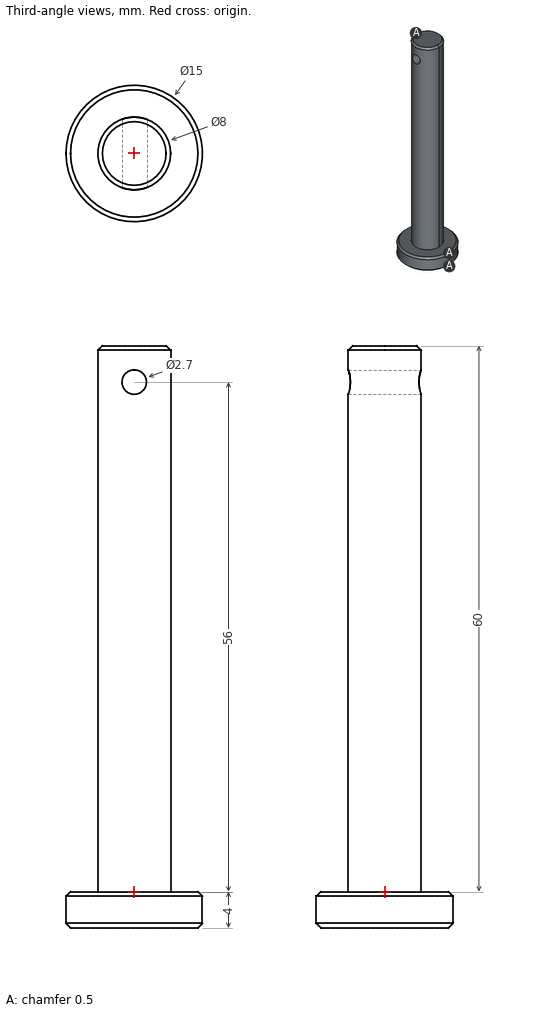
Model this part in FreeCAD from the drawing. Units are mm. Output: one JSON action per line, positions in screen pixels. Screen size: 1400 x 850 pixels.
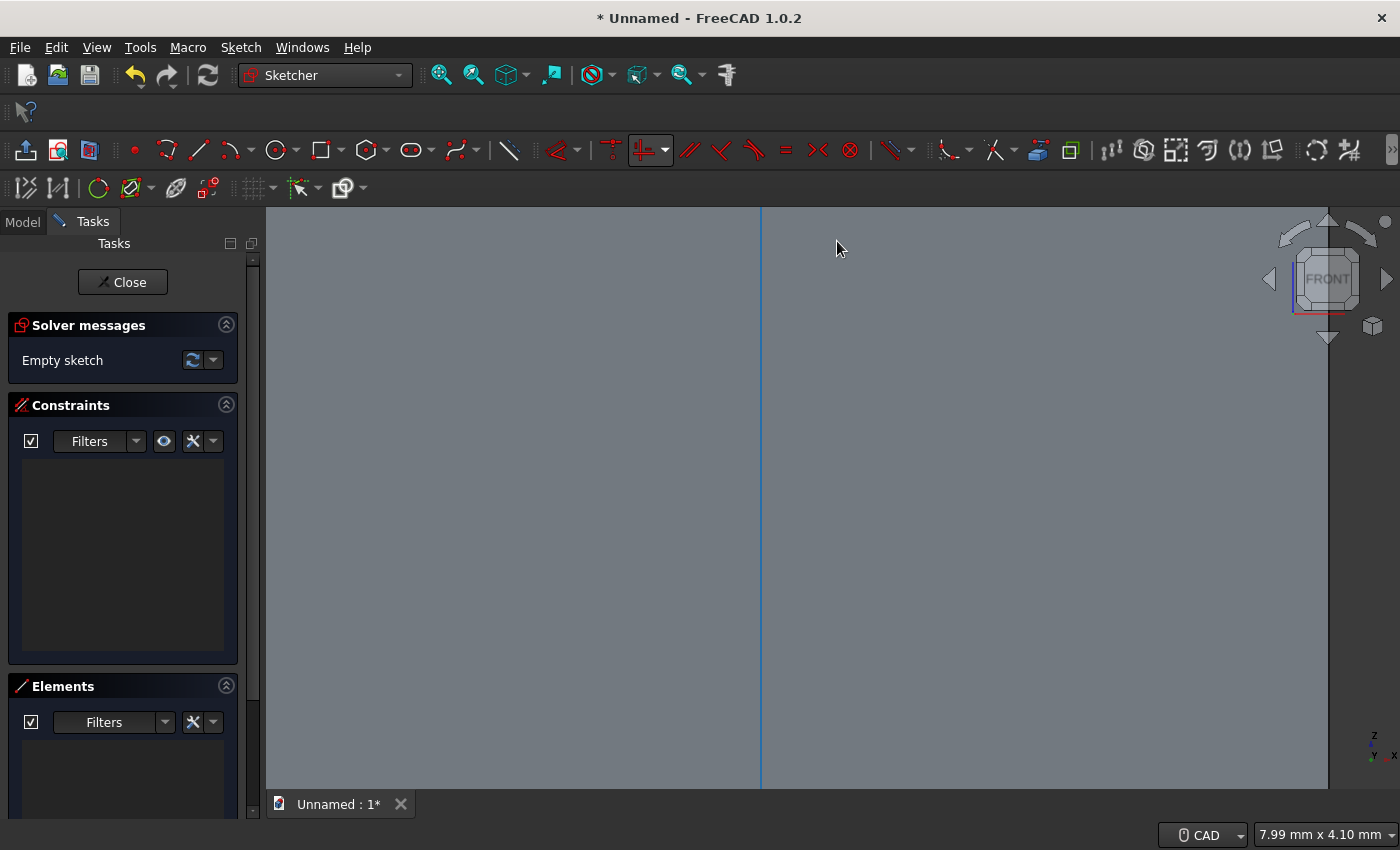
{"action": "left_click", "coordinate": [276, 150]}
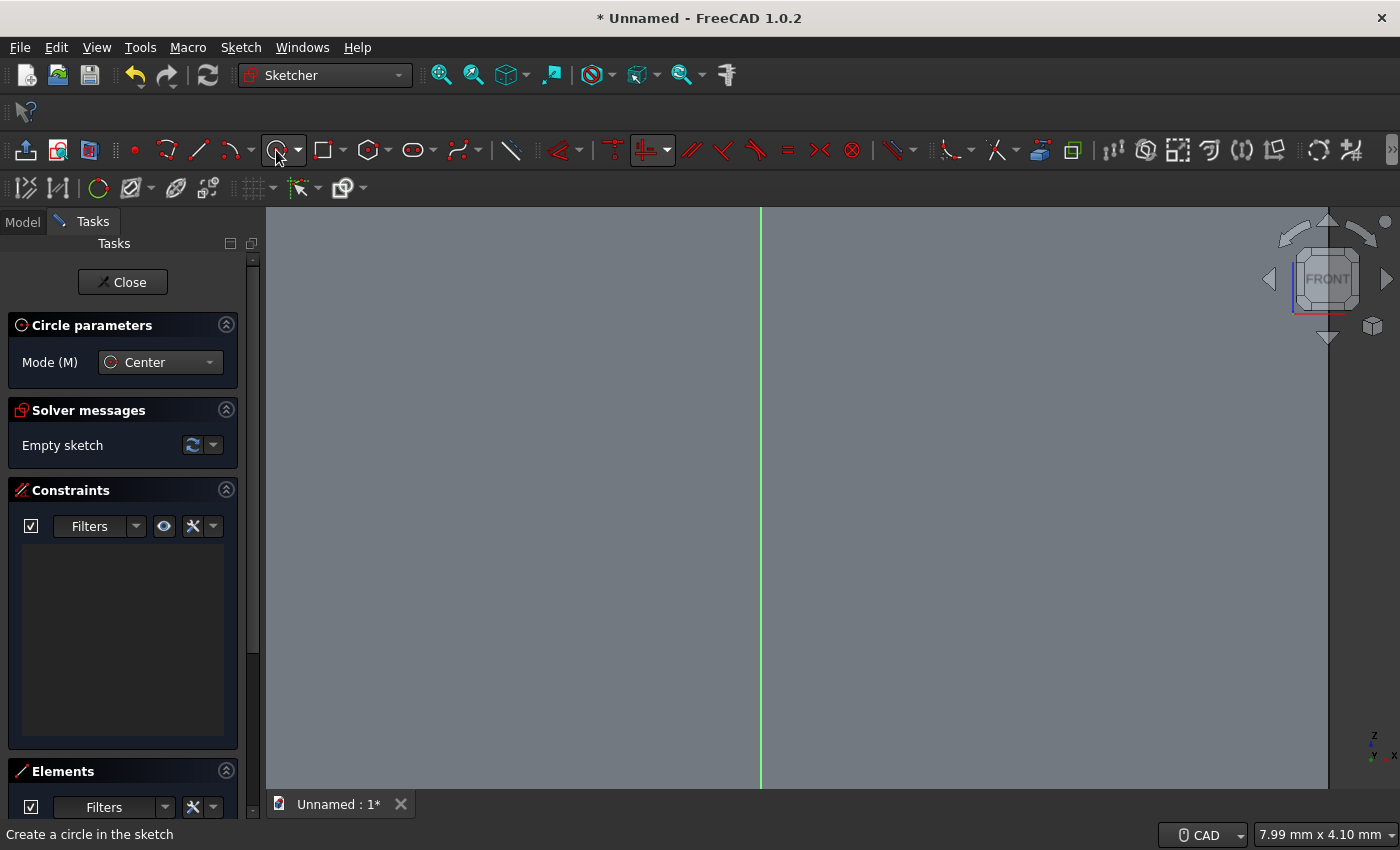
{"action": "left_click", "coordinate": [761, 491]}
{"action": "left_click", "coordinate": [897, 356]}
{"action": "key", "text": "Escape"}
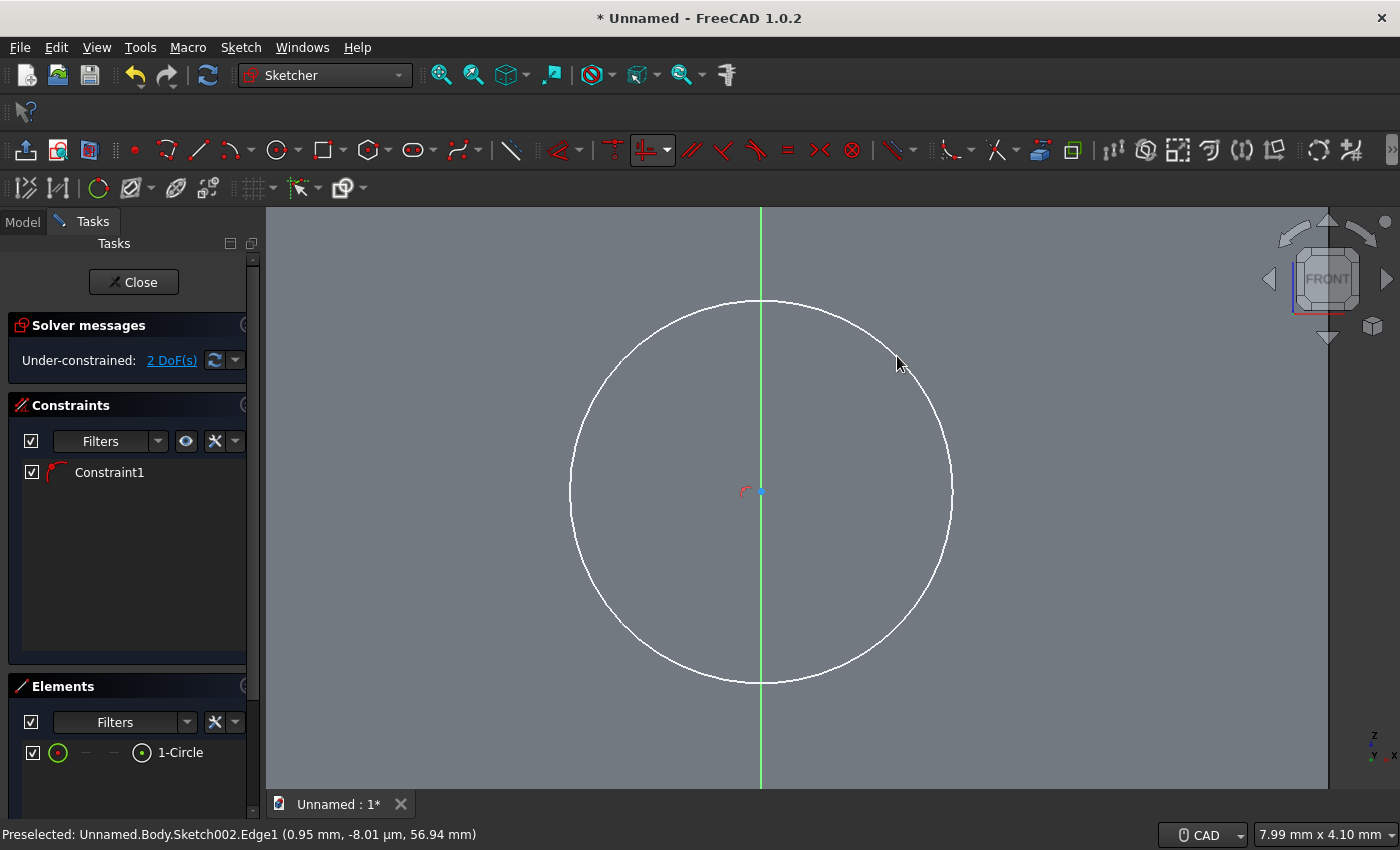
{"action": "left_click", "coordinate": [558, 150]}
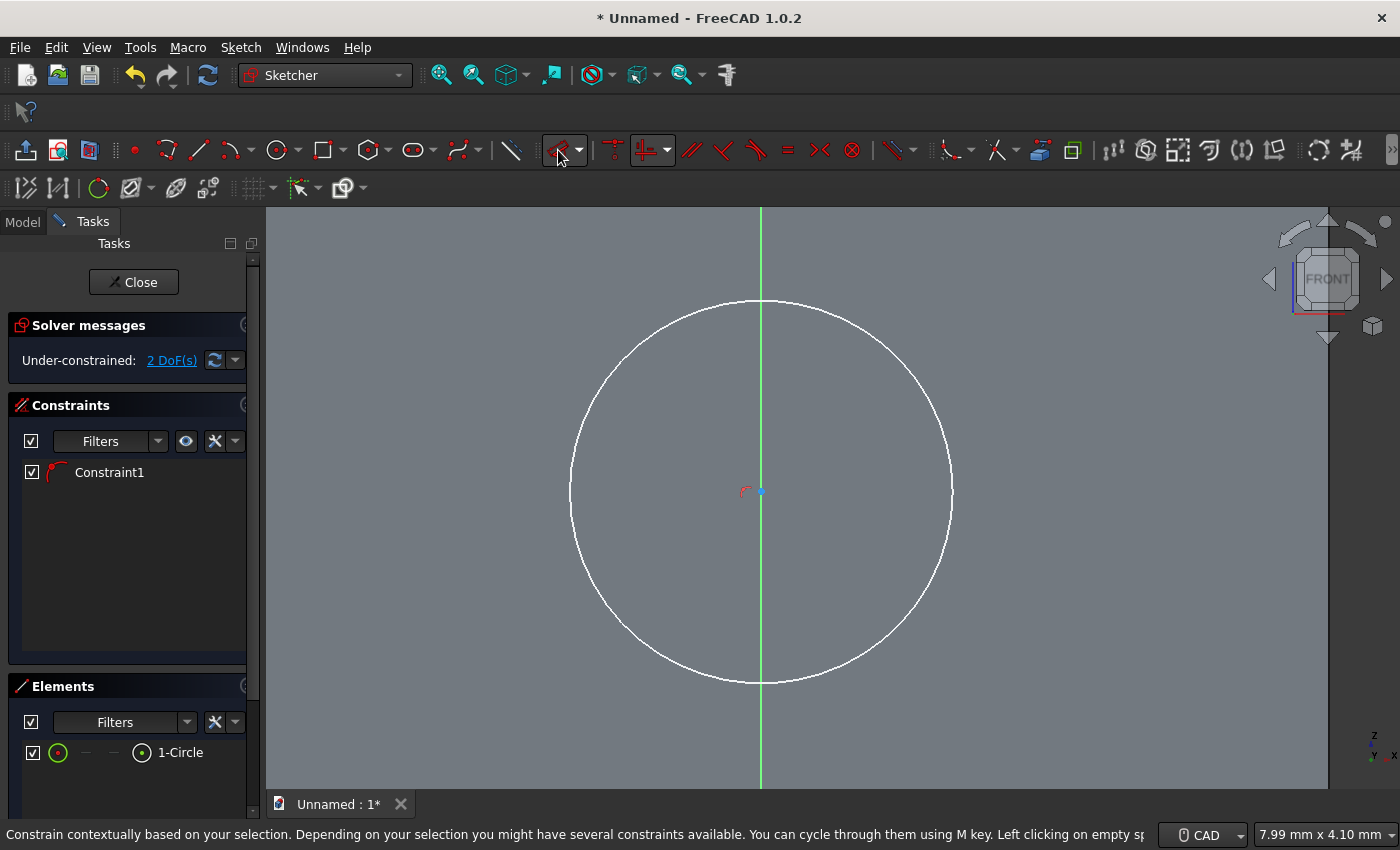
{"action": "left_click", "coordinate": [896, 356]}
{"action": "left_click", "coordinate": [919, 333]}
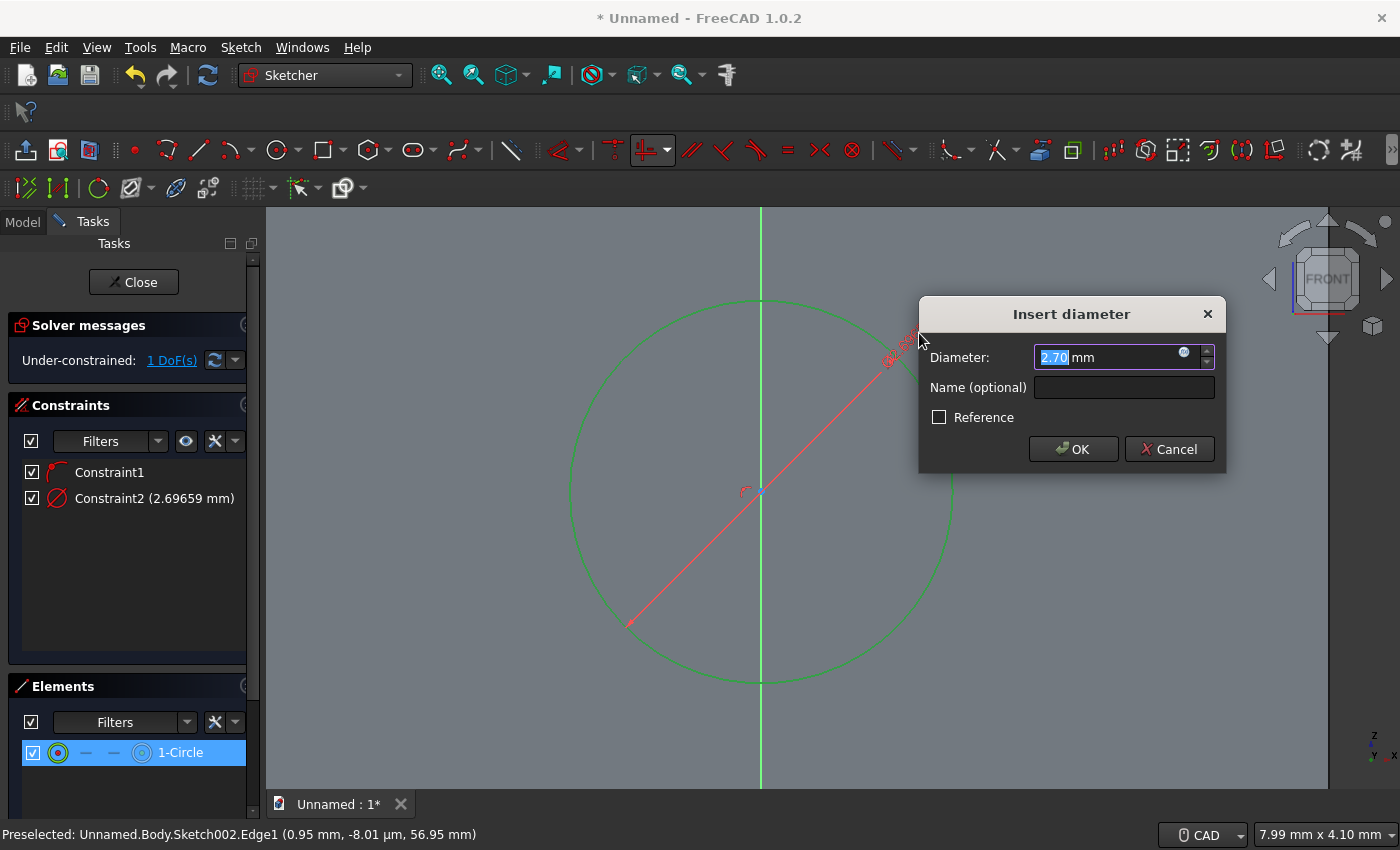
{"action": "type", "text": "2.7"}
{"action": "key", "text": "Return"}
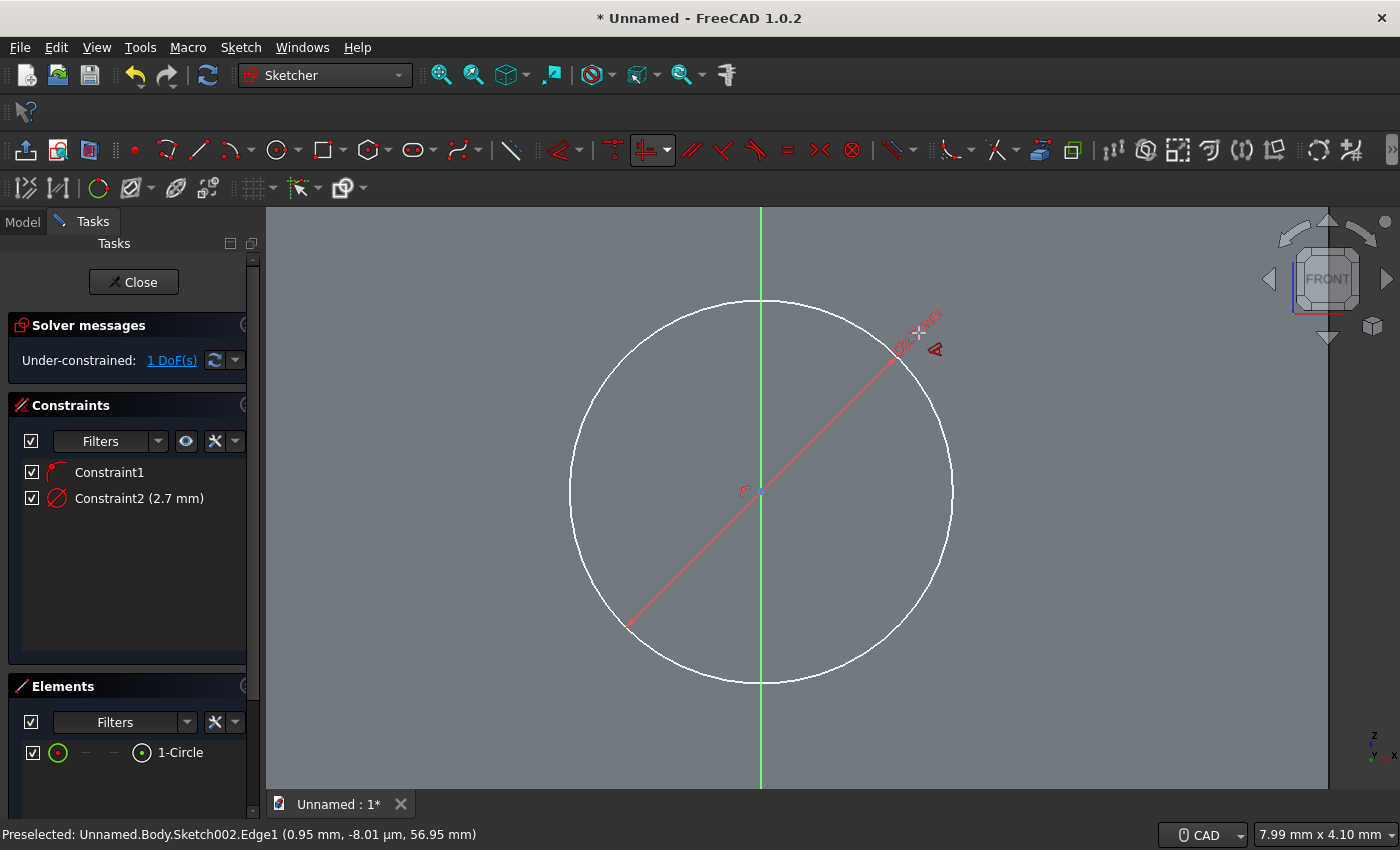
{"action": "left_click", "coordinate": [761, 492]}
{"action": "left_click", "coordinate": [795, 626]}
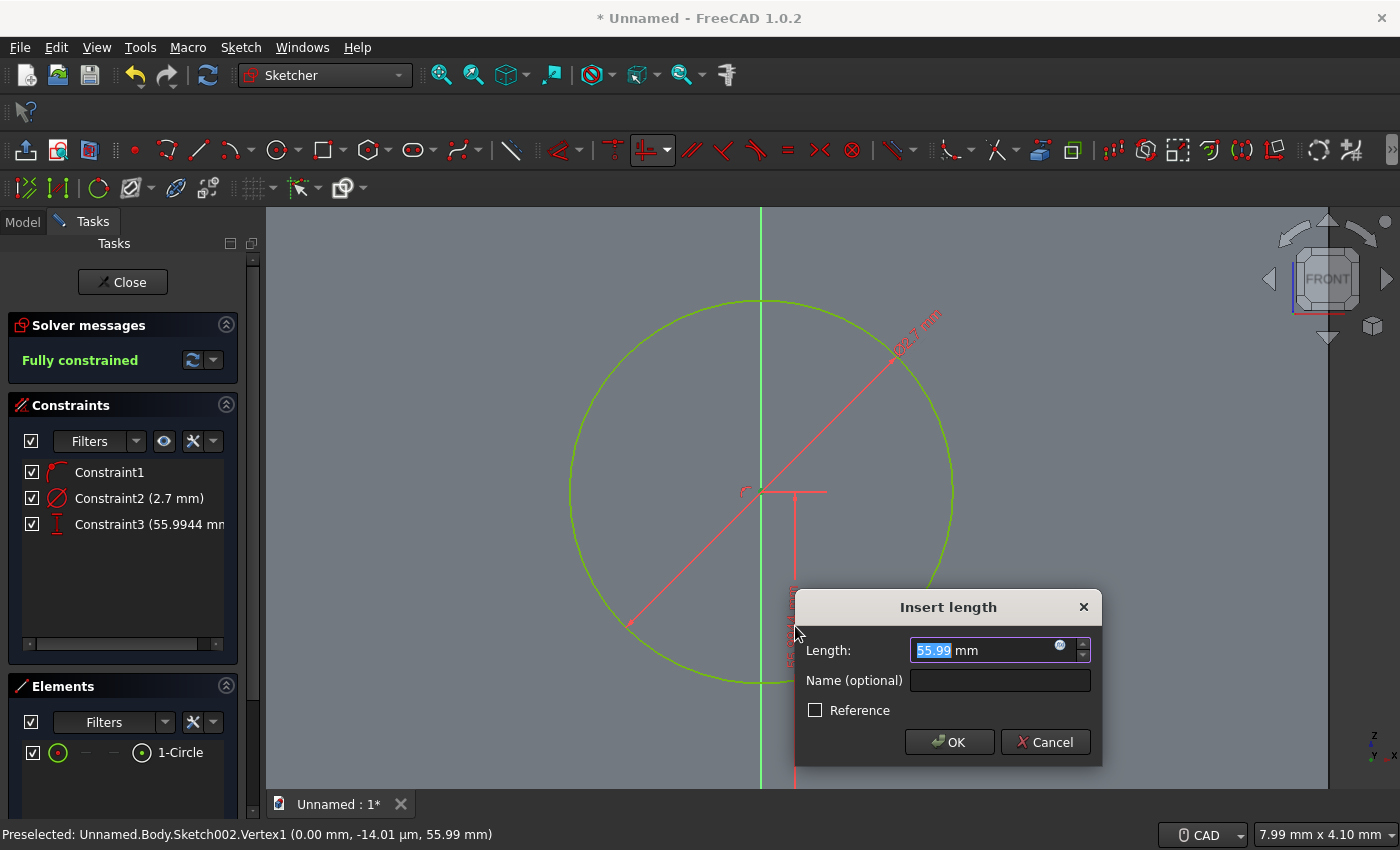
{"action": "type", "text": "56"}
{"action": "key", "text": "Return"}
{"action": "key", "text": "Escape"}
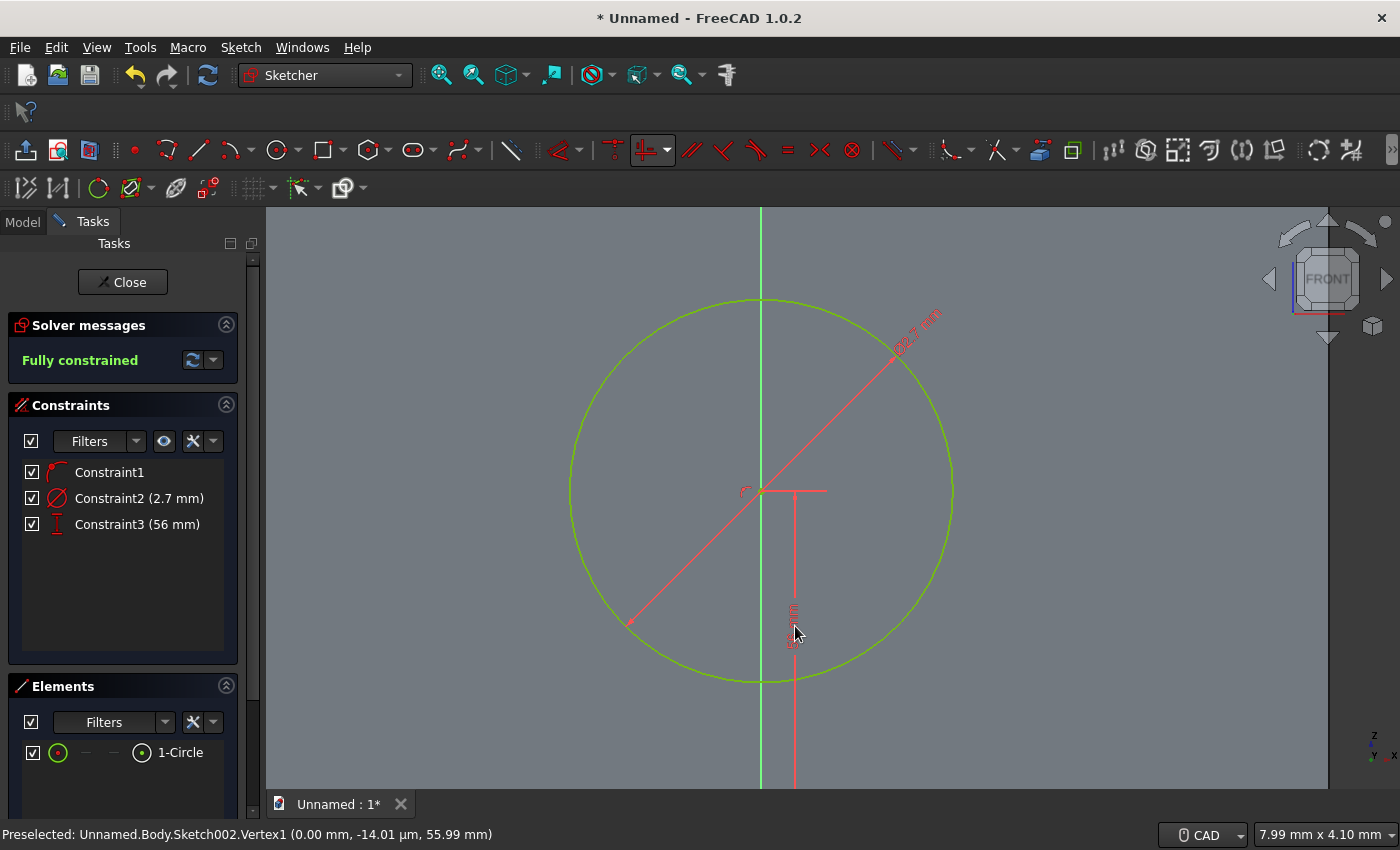
{"action": "left_click", "coordinate": [123, 282]}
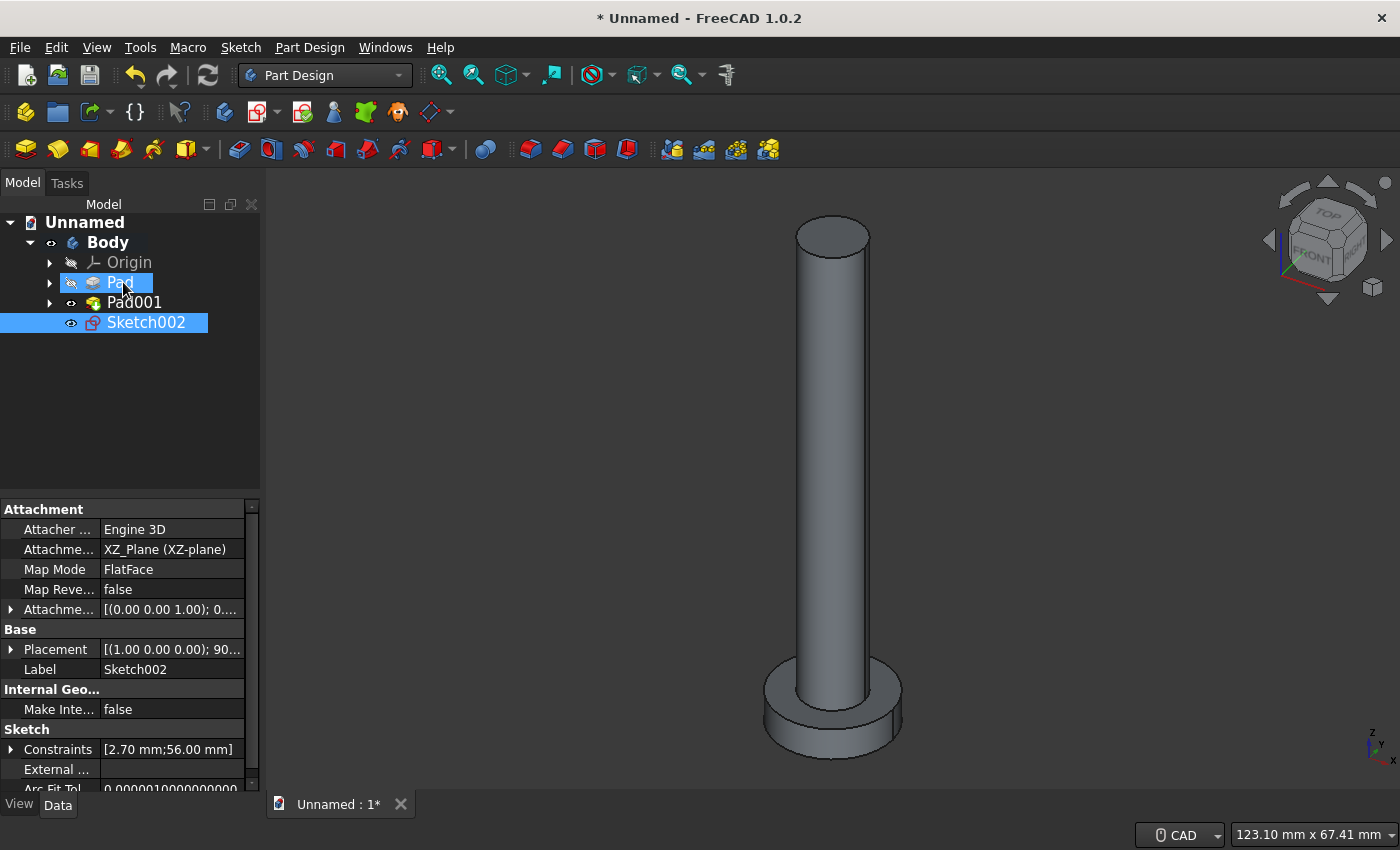
{"action": "left_click", "coordinate": [240, 150]}